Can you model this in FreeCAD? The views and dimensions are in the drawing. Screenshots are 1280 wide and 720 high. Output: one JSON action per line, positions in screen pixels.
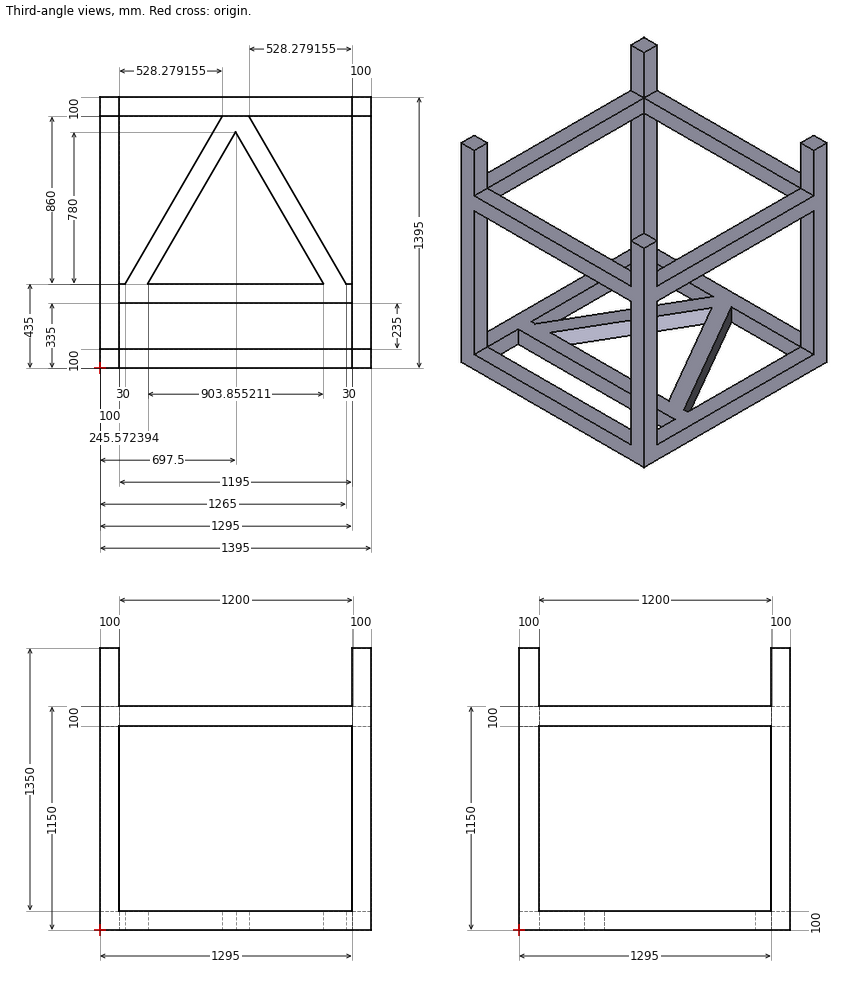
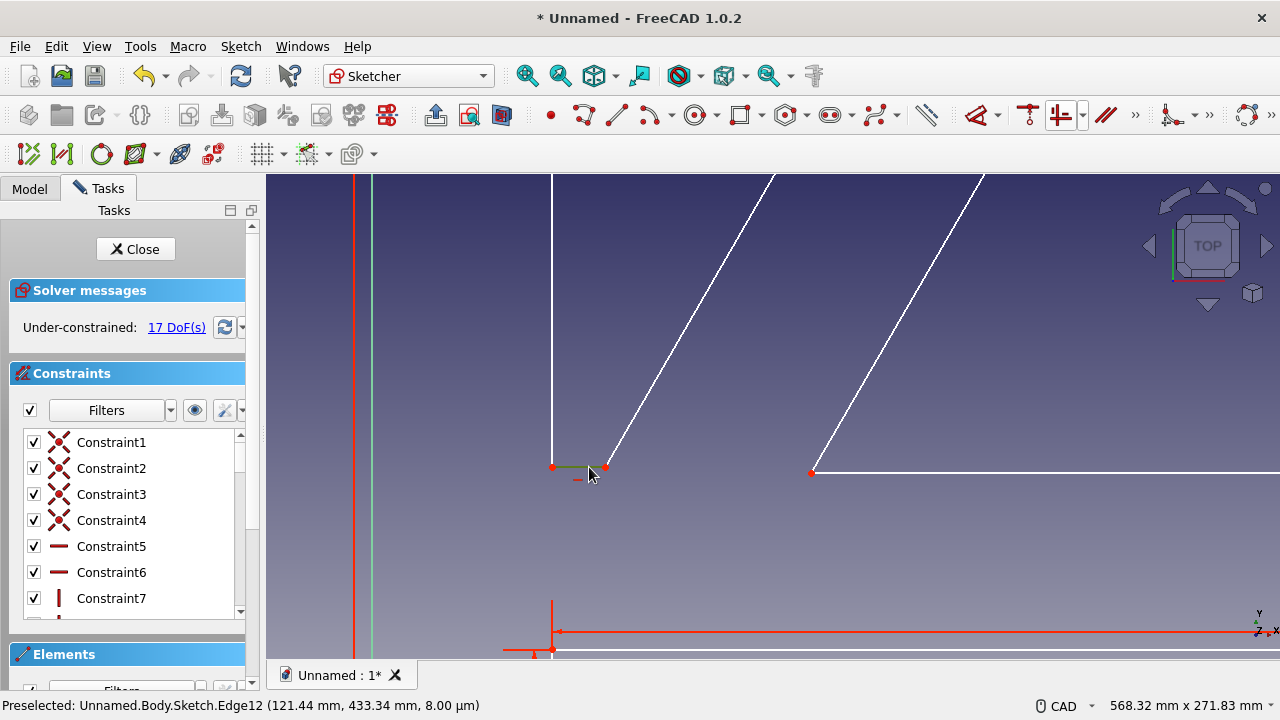
{"action": "key", "text": "l"}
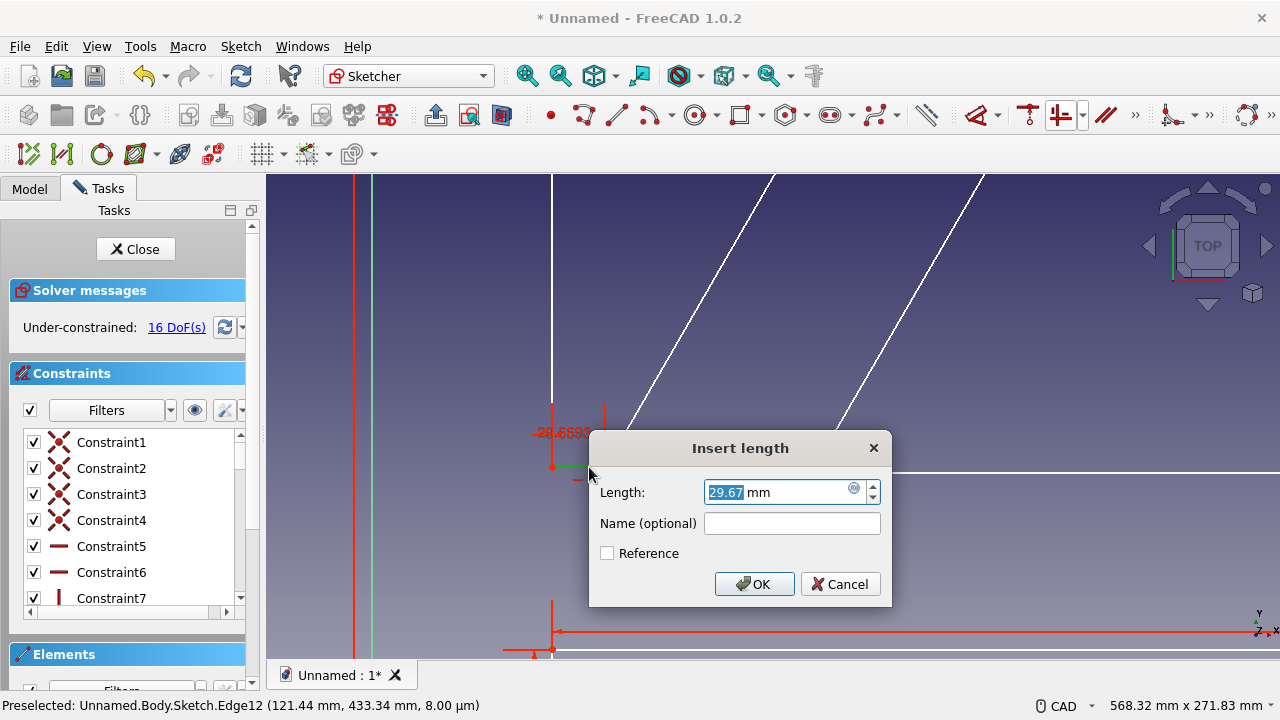
{"action": "type", "text": "30"}
{"action": "key", "text": "Return"}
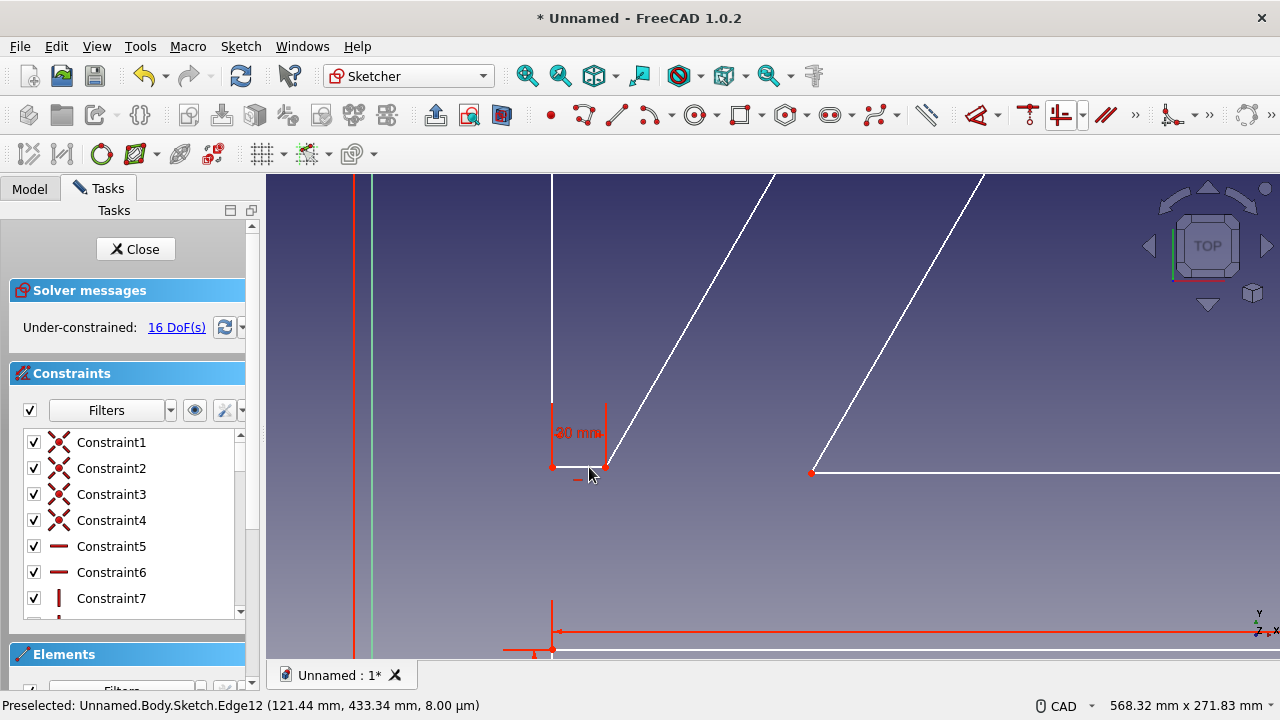
{"action": "scroll", "coordinate": [591, 469], "scroll_direction": "down", "scroll_amount": 11}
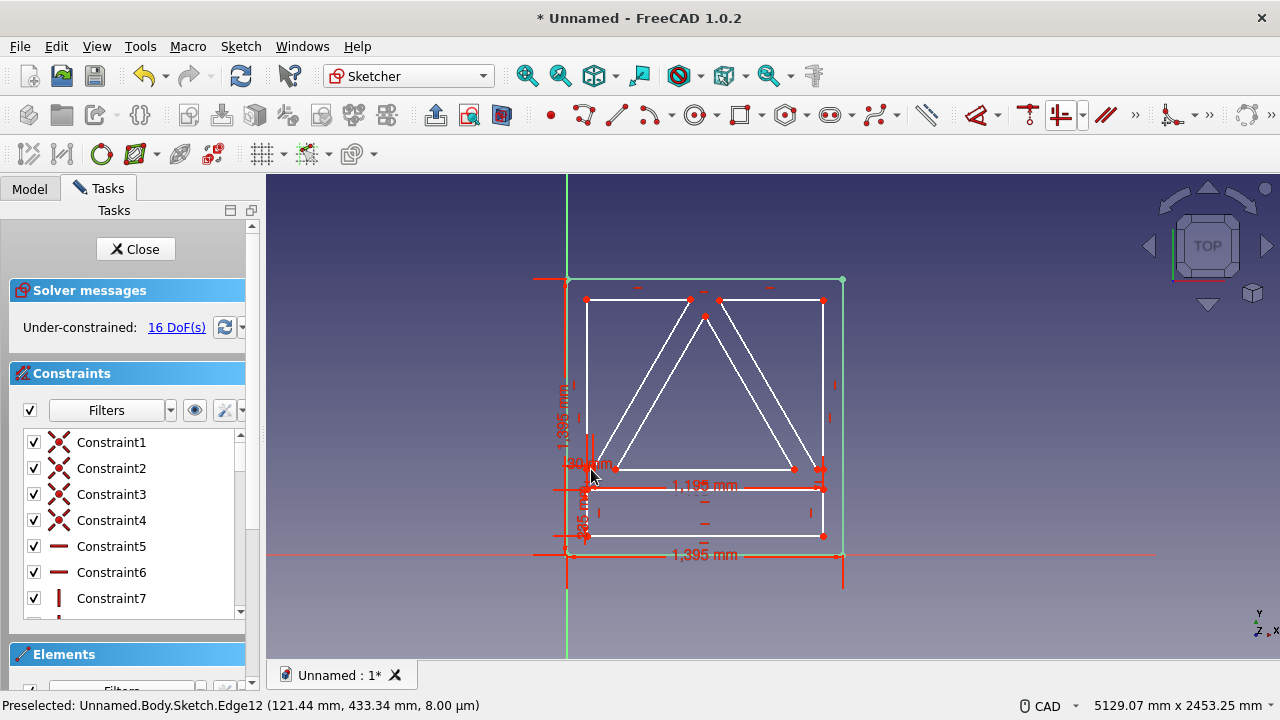
{"action": "scroll", "coordinate": [821, 469], "scroll_direction": "up", "scroll_amount": 11}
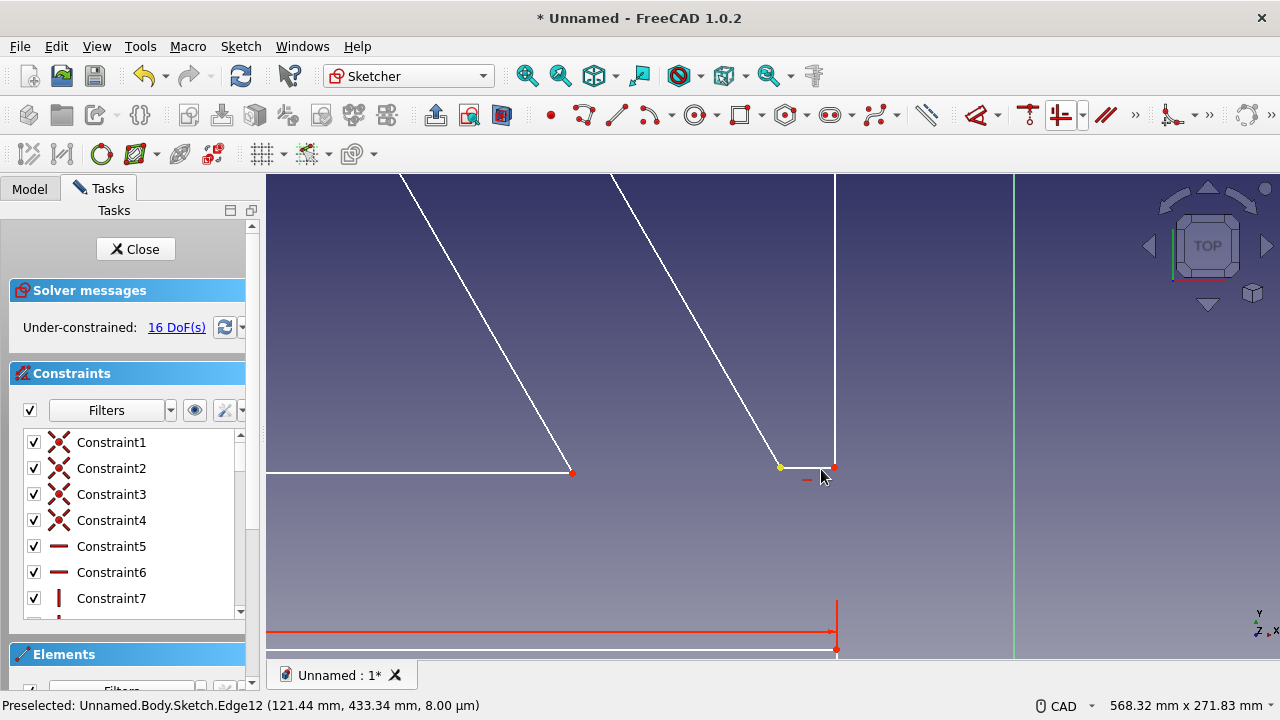
{"action": "left_click", "coordinate": [818, 468]}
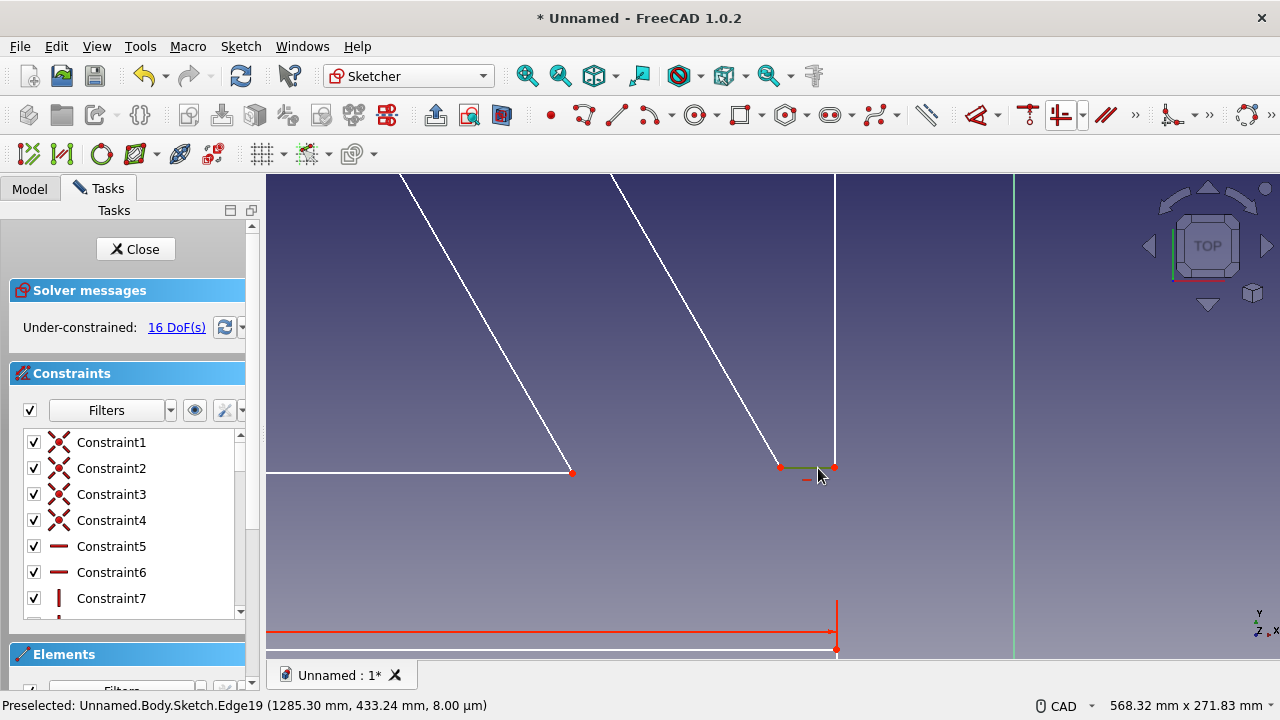
{"action": "left_click", "coordinate": [998, 116]}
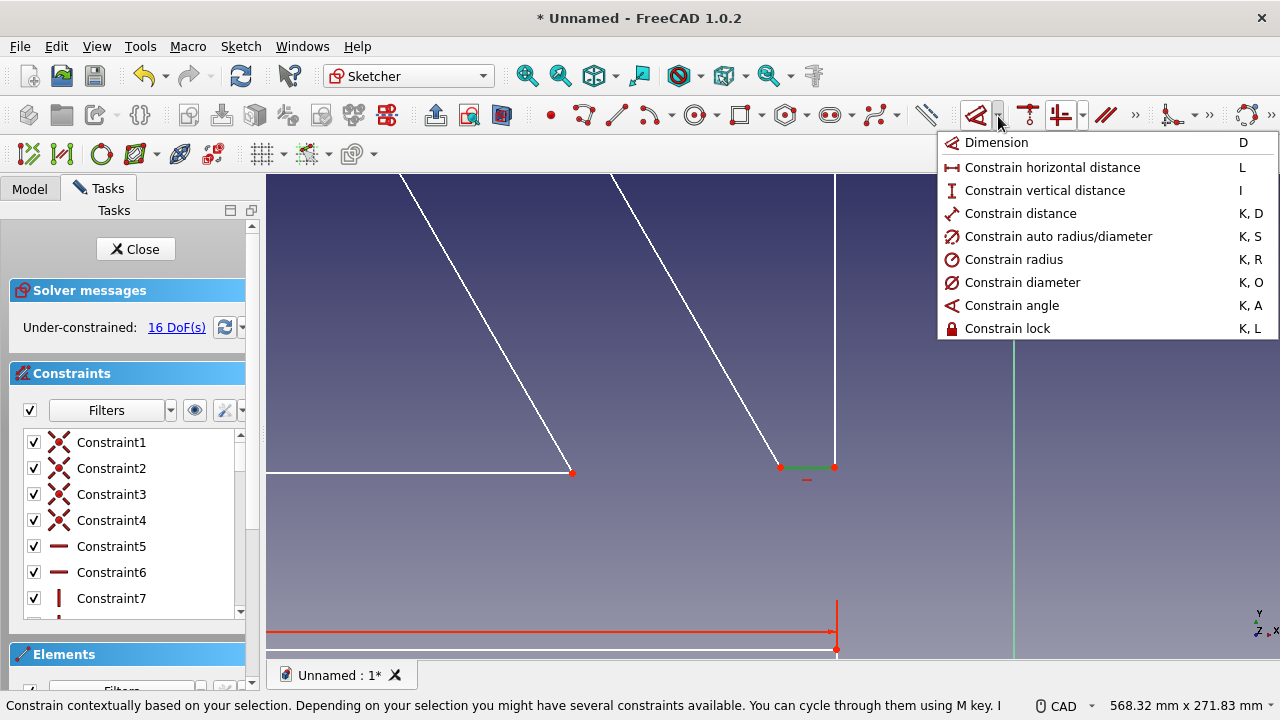
{"action": "left_click", "coordinate": [1108, 168]}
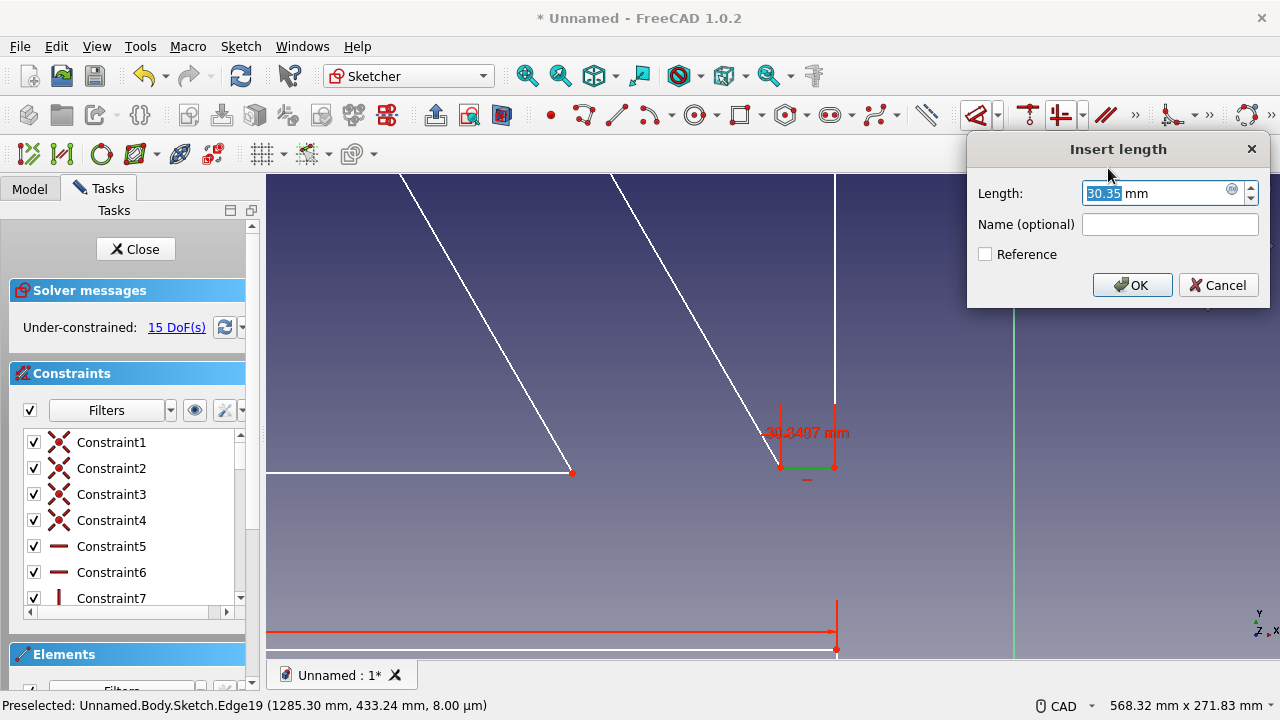
{"action": "type", "text": "30"}
{"action": "key", "text": "Return"}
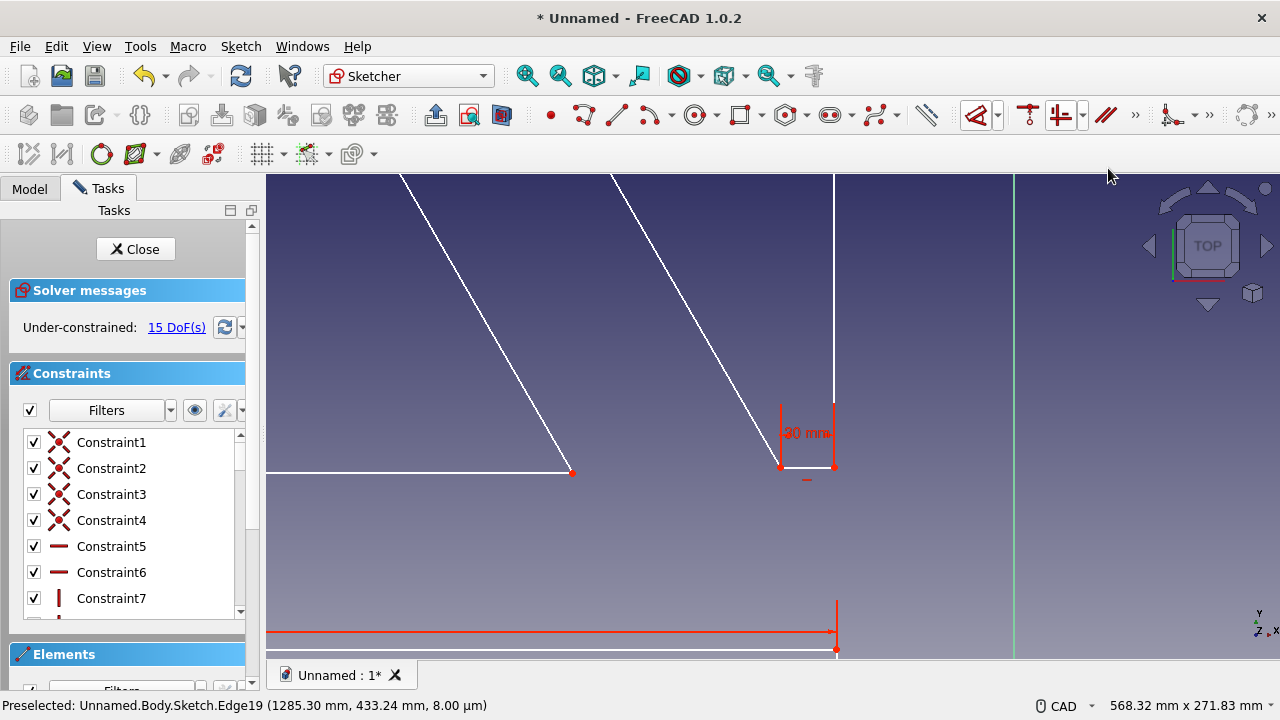
{"action": "scroll", "coordinate": [821, 469], "scroll_direction": "down", "scroll_amount": 11}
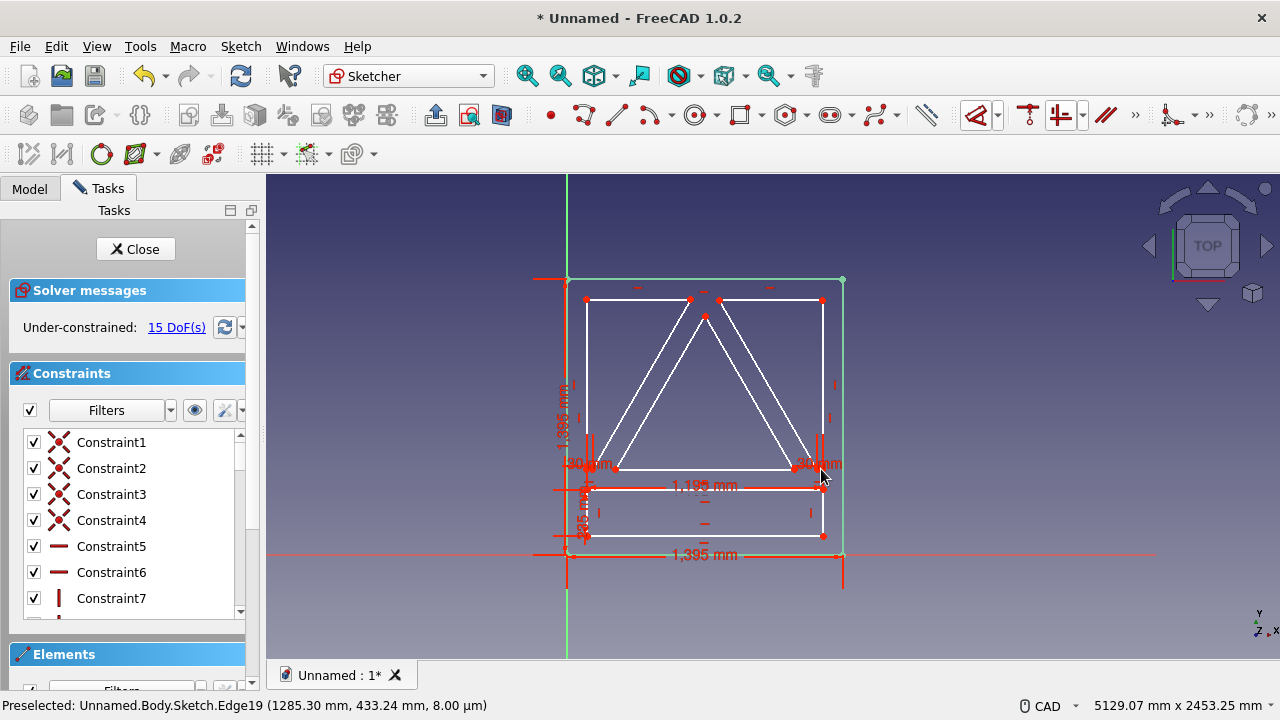
{"action": "left_click", "coordinate": [587, 418]}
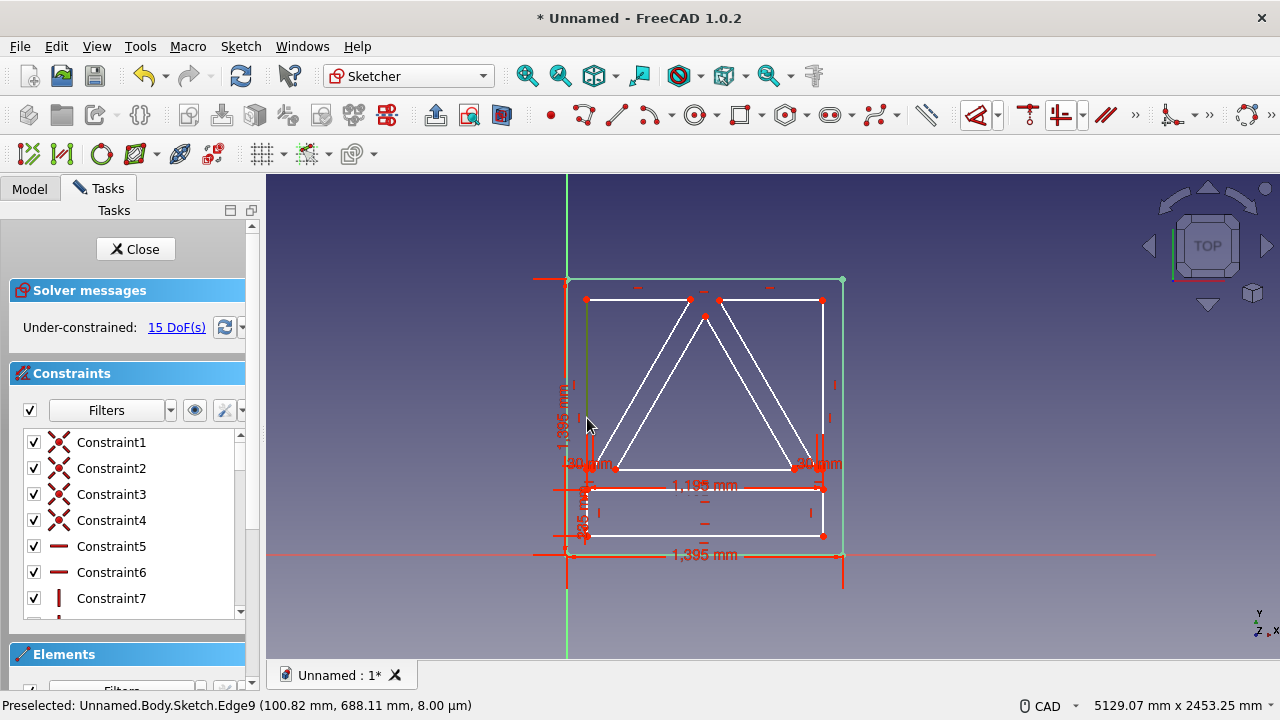
{"action": "left_click", "coordinate": [998, 116]}